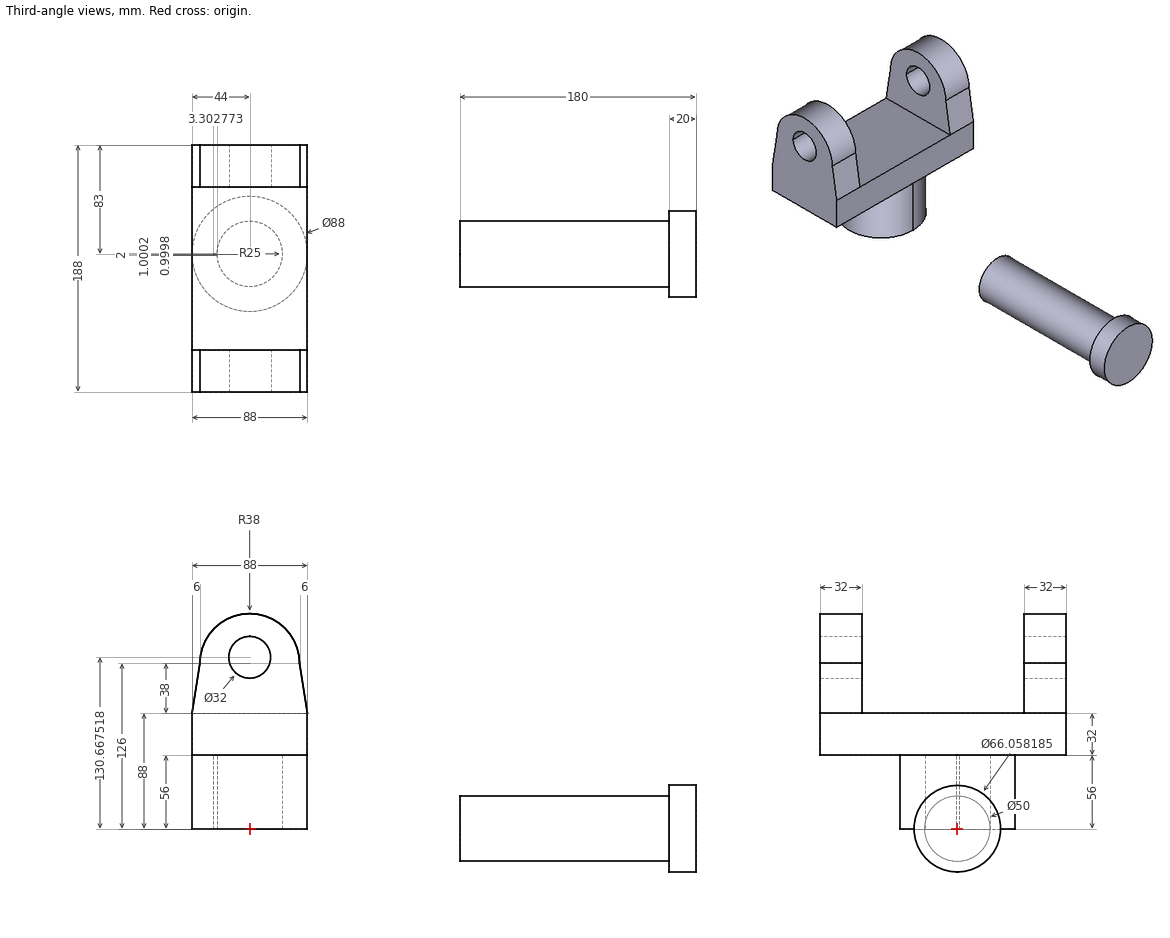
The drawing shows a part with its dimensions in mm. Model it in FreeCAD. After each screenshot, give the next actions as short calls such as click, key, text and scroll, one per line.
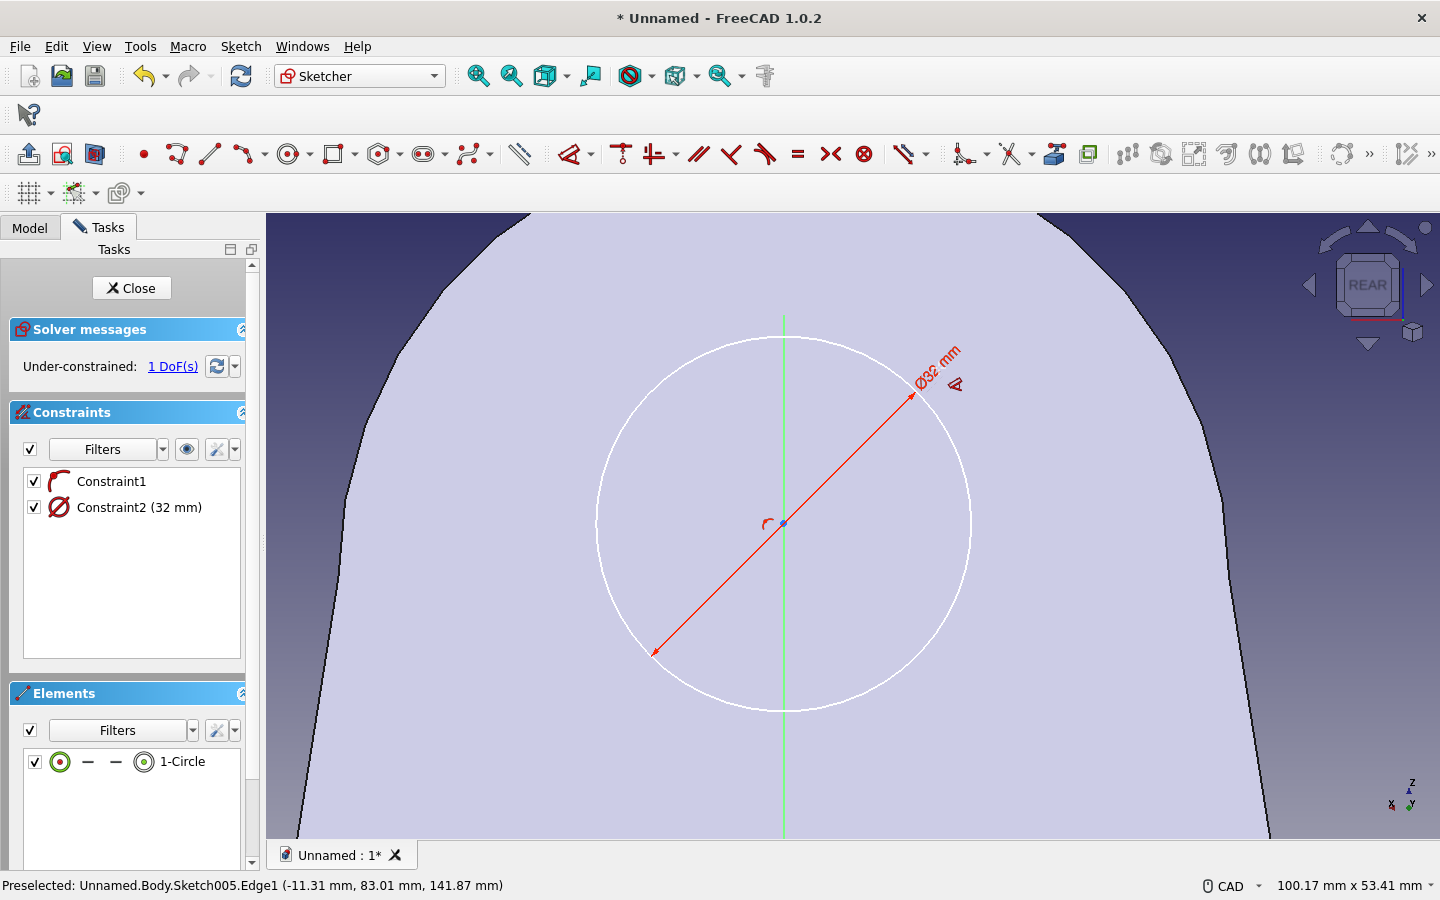
click(784, 524)
click(818, 668)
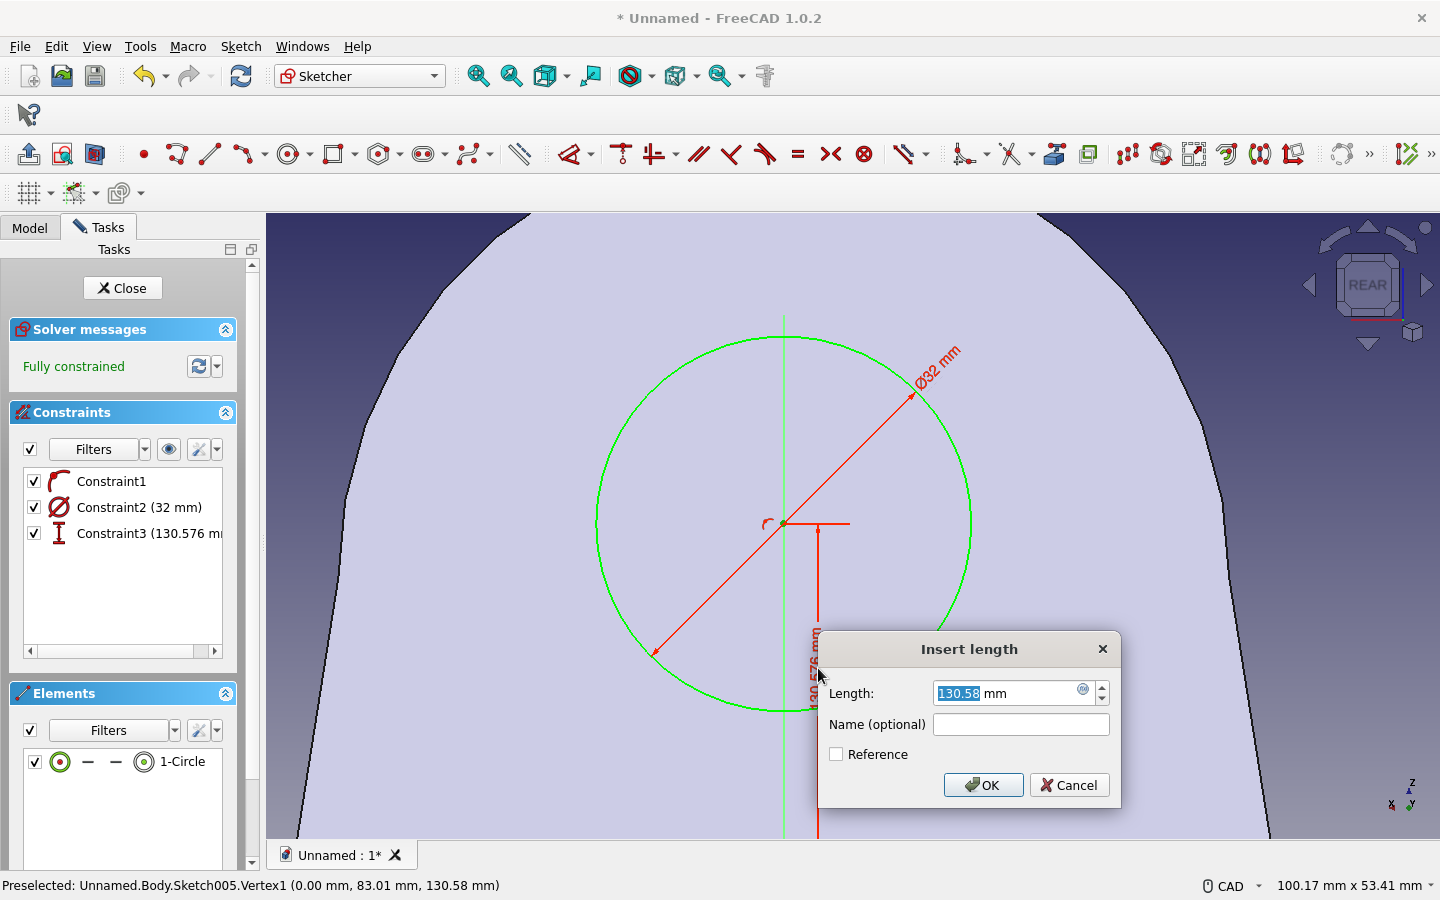
text(130.667518)
key(Return)
key(Escape)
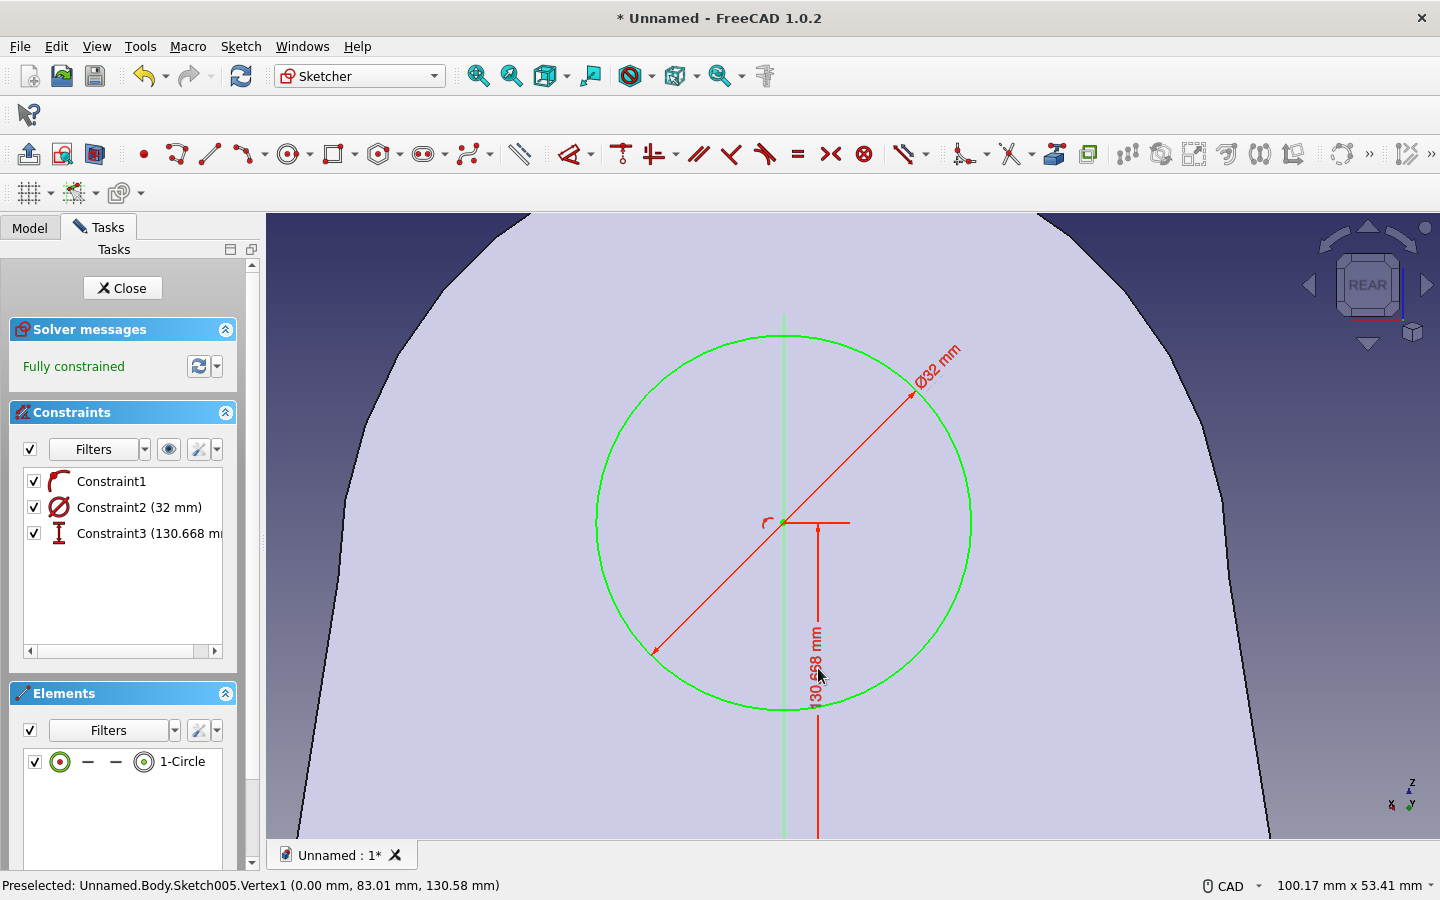
click(123, 288)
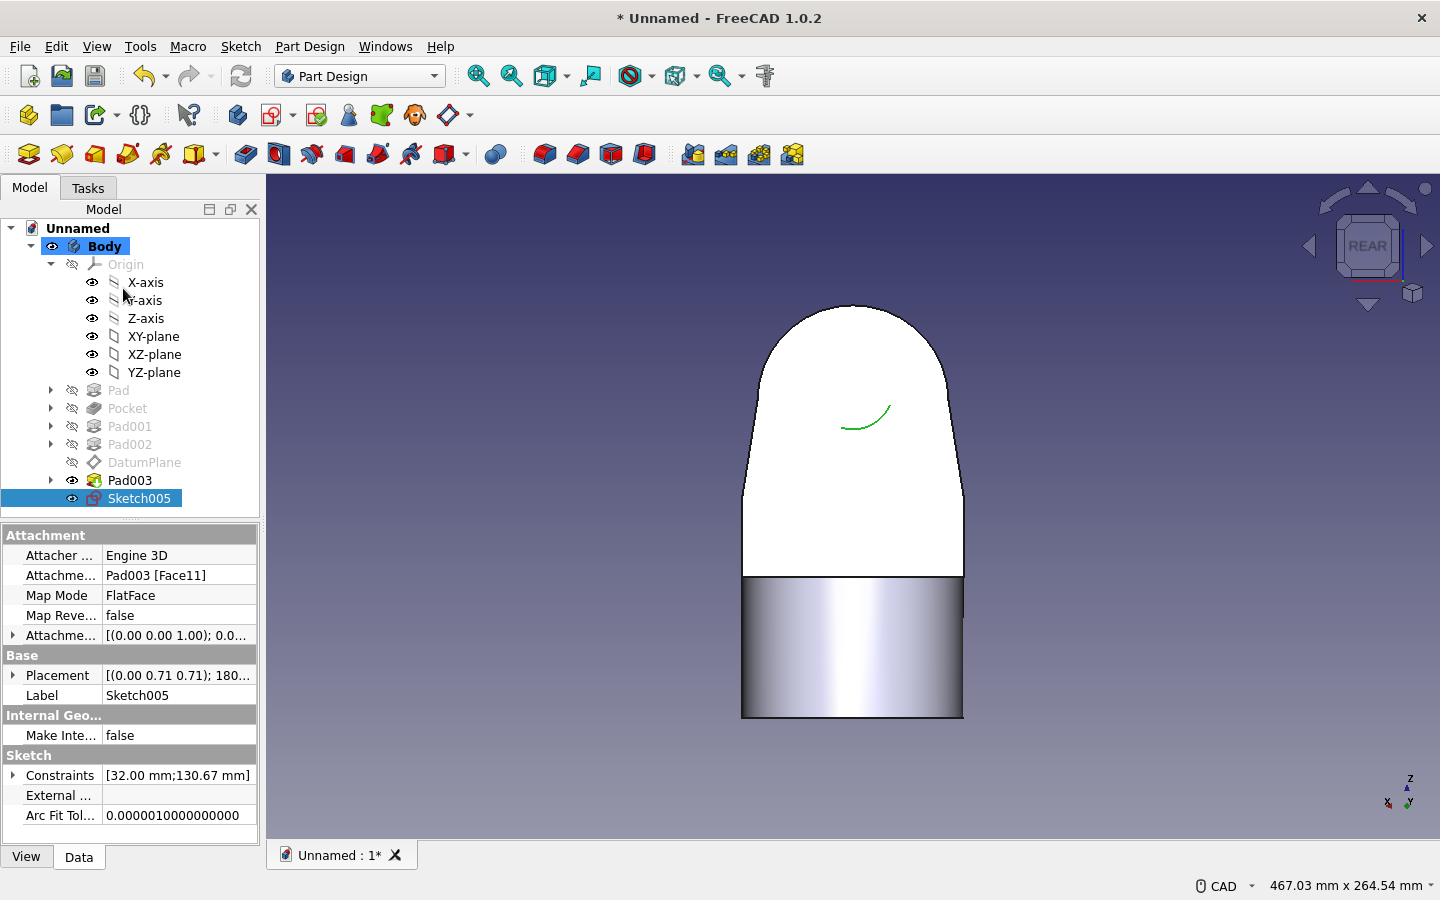
click(246, 154)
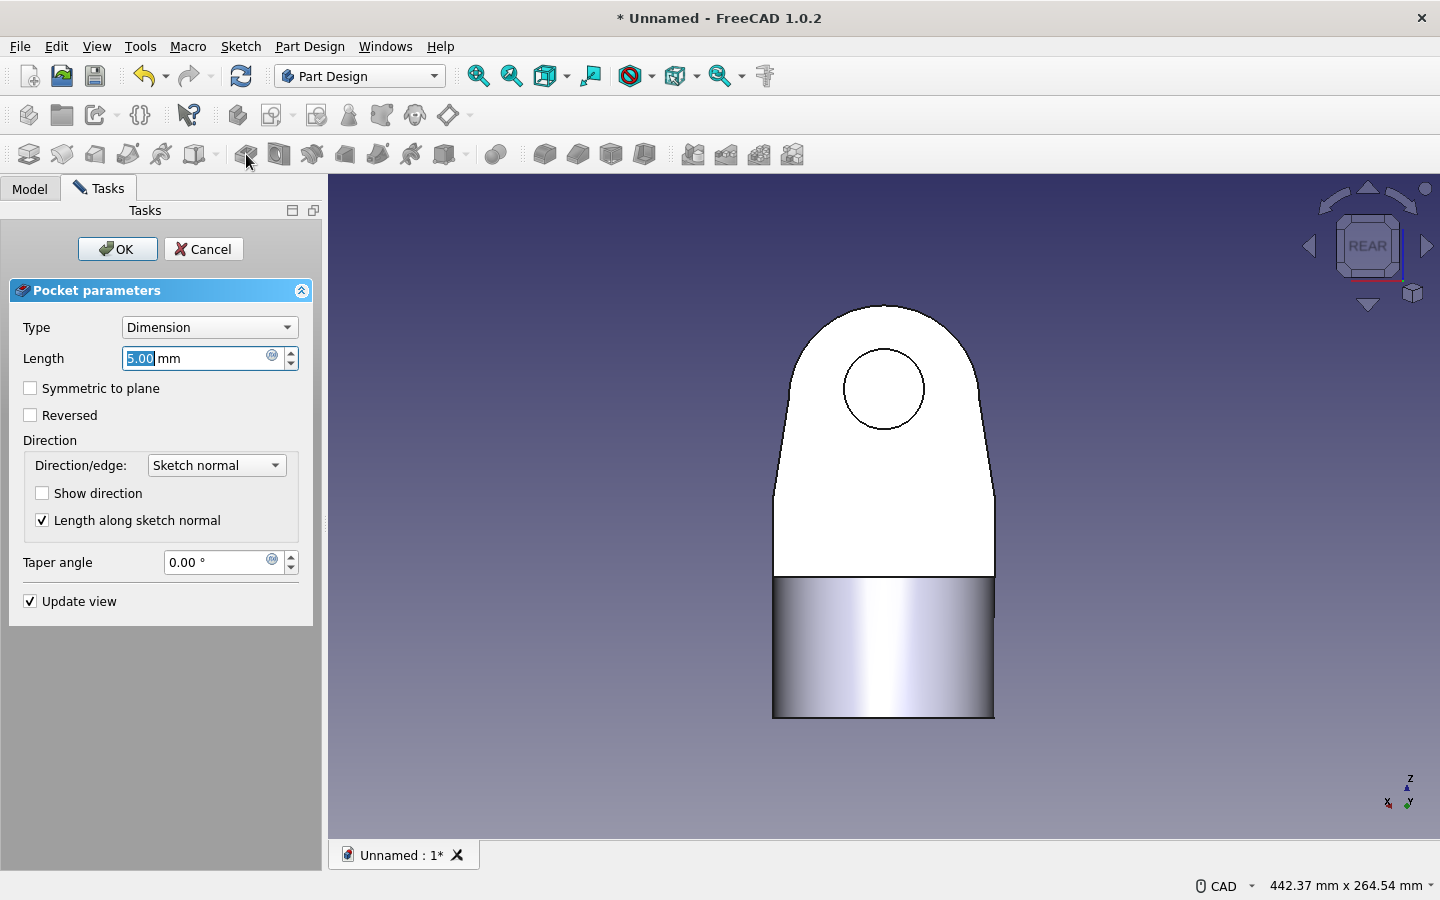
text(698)
key(Tab)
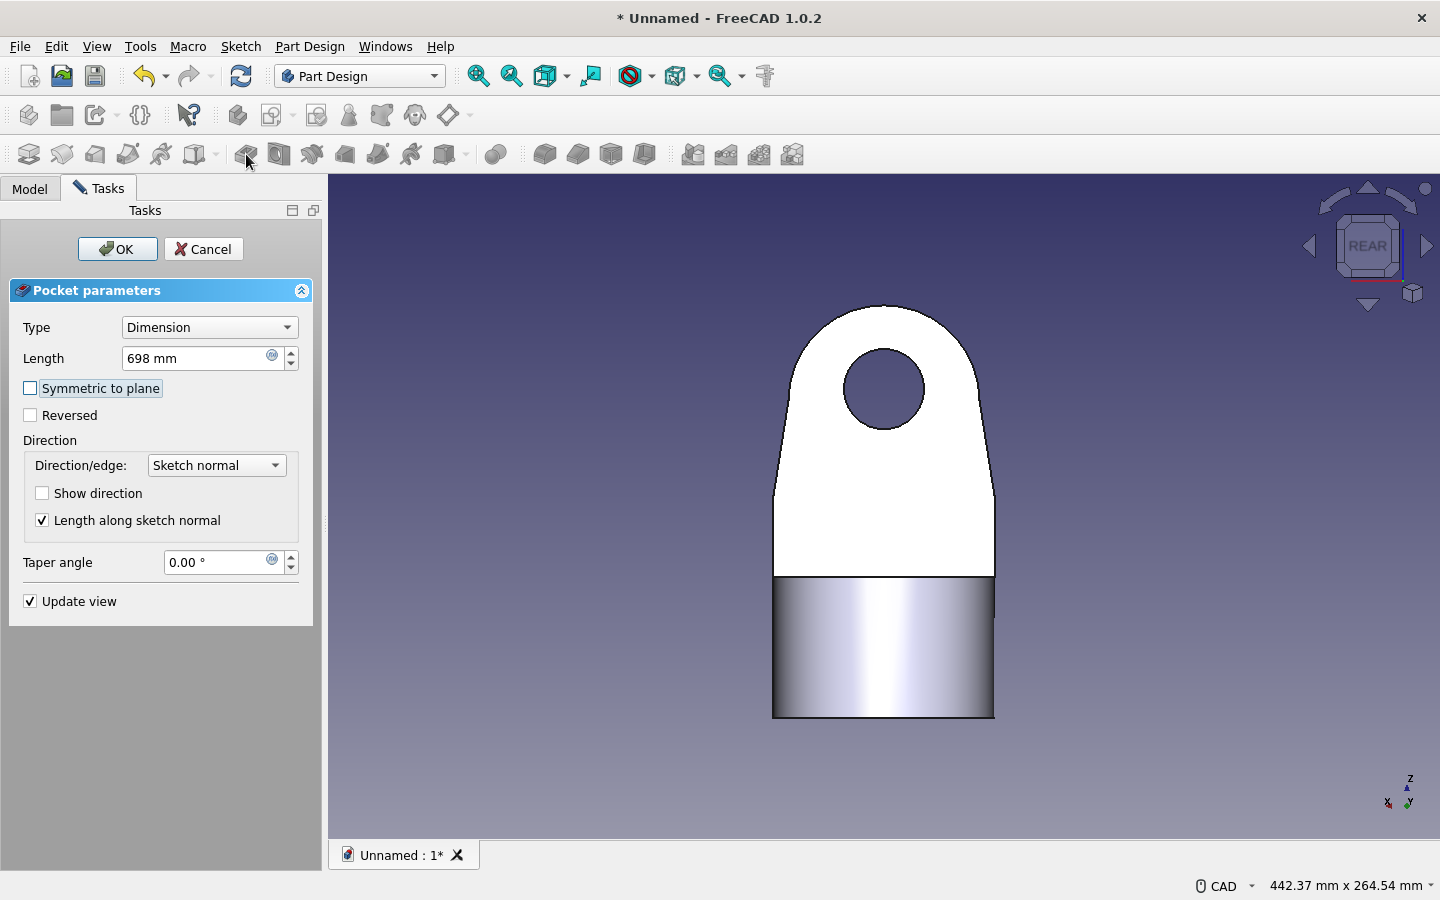
click(118, 249)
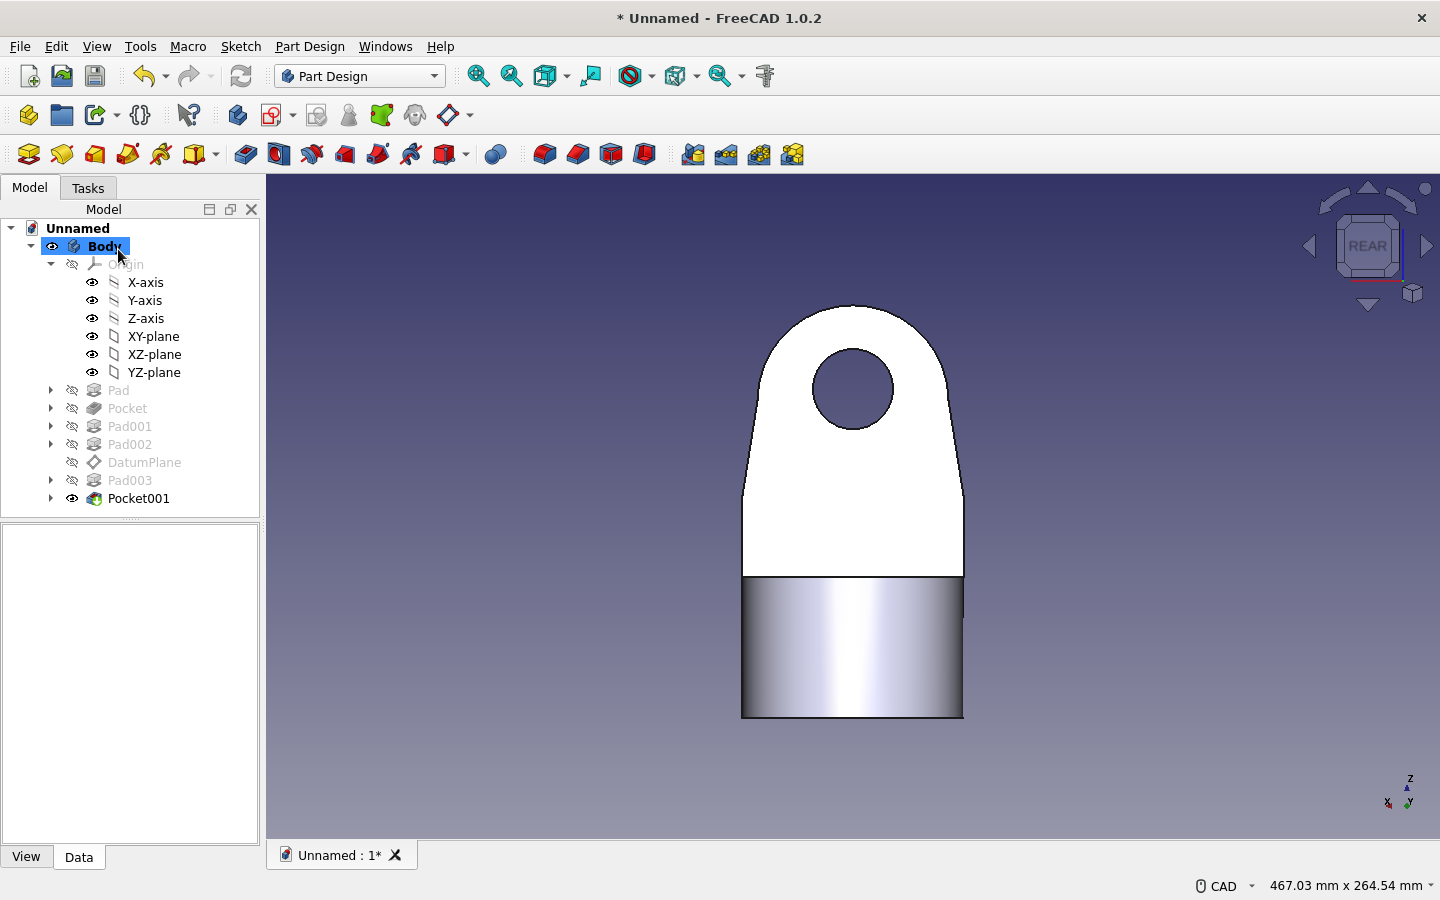
click(238, 116)